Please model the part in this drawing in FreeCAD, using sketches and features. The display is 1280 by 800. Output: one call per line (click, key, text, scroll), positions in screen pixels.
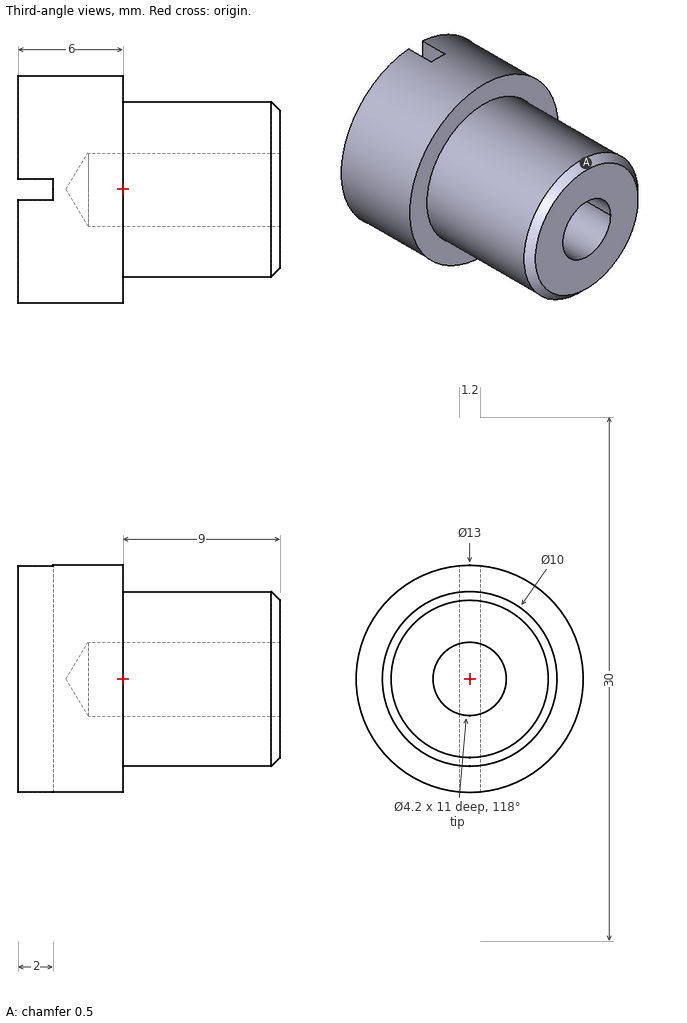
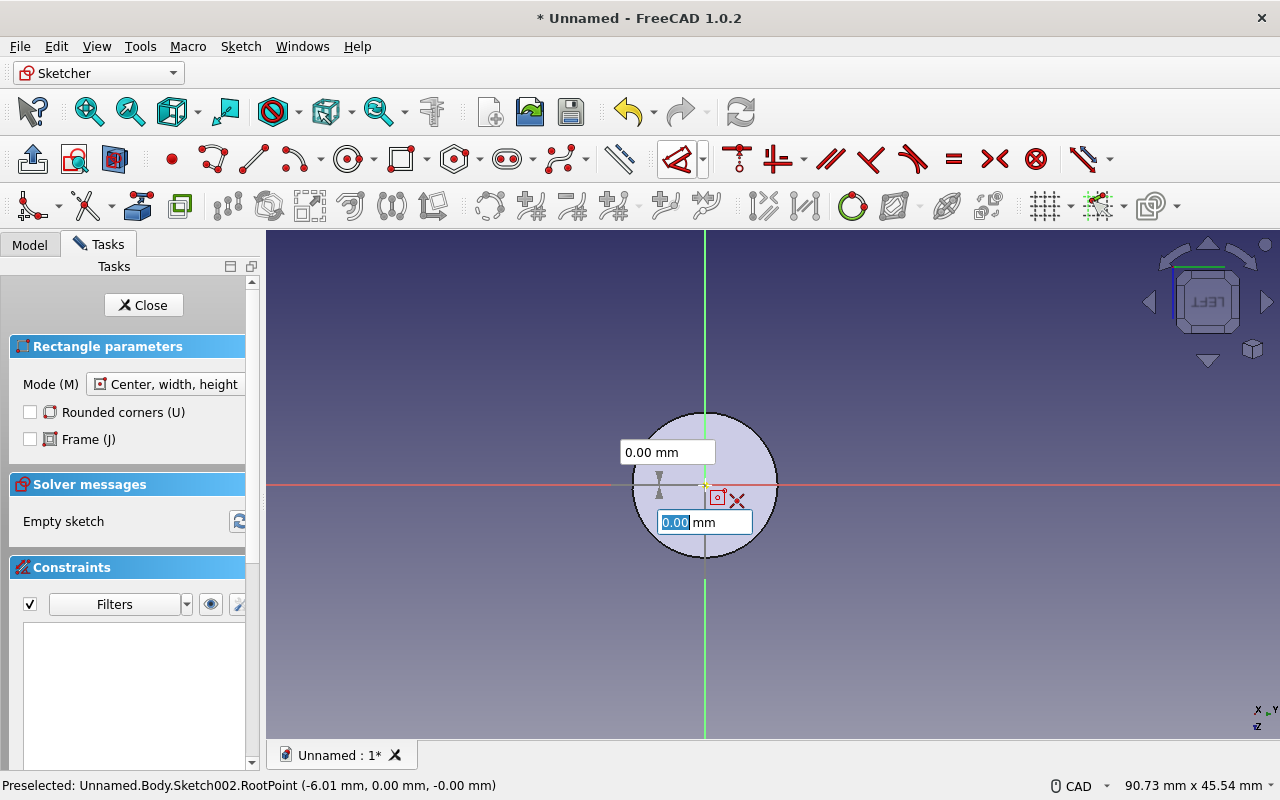
scroll(712, 317, up, 5)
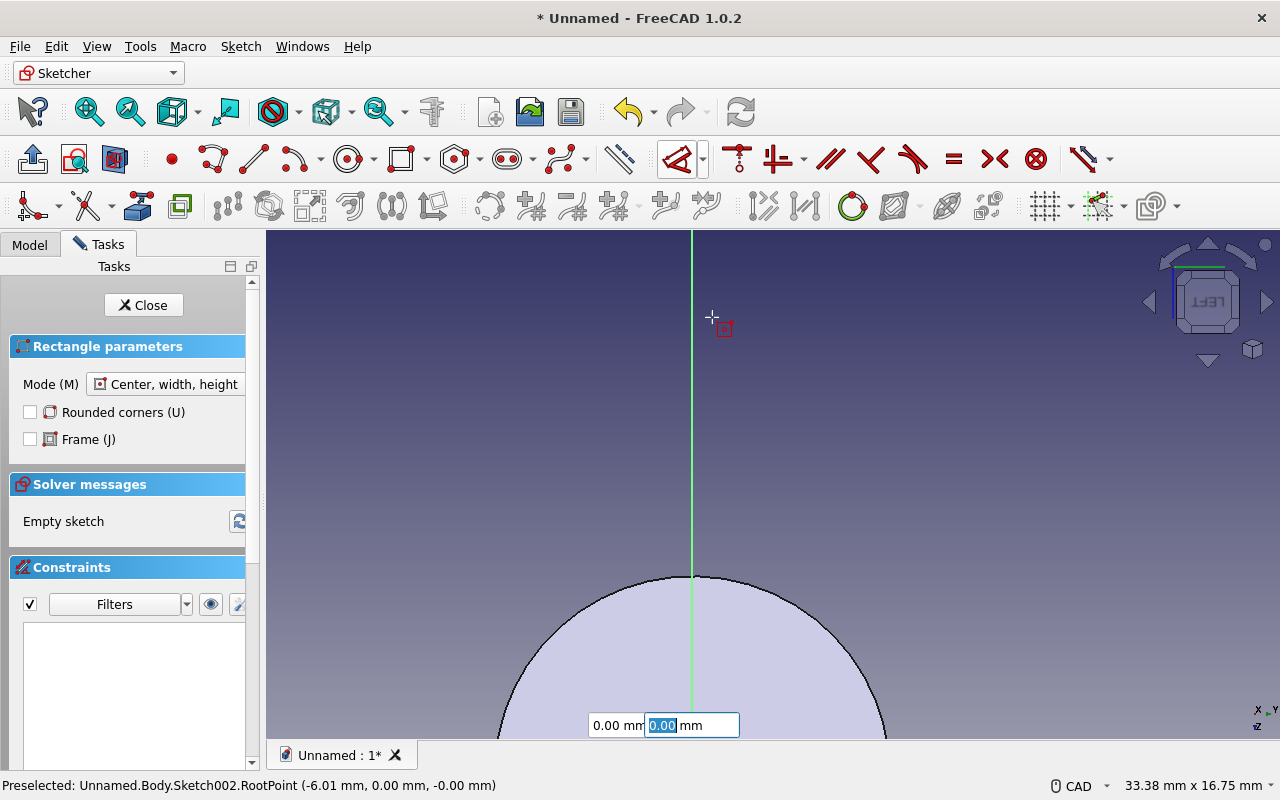
click(710, 318)
key(Escape)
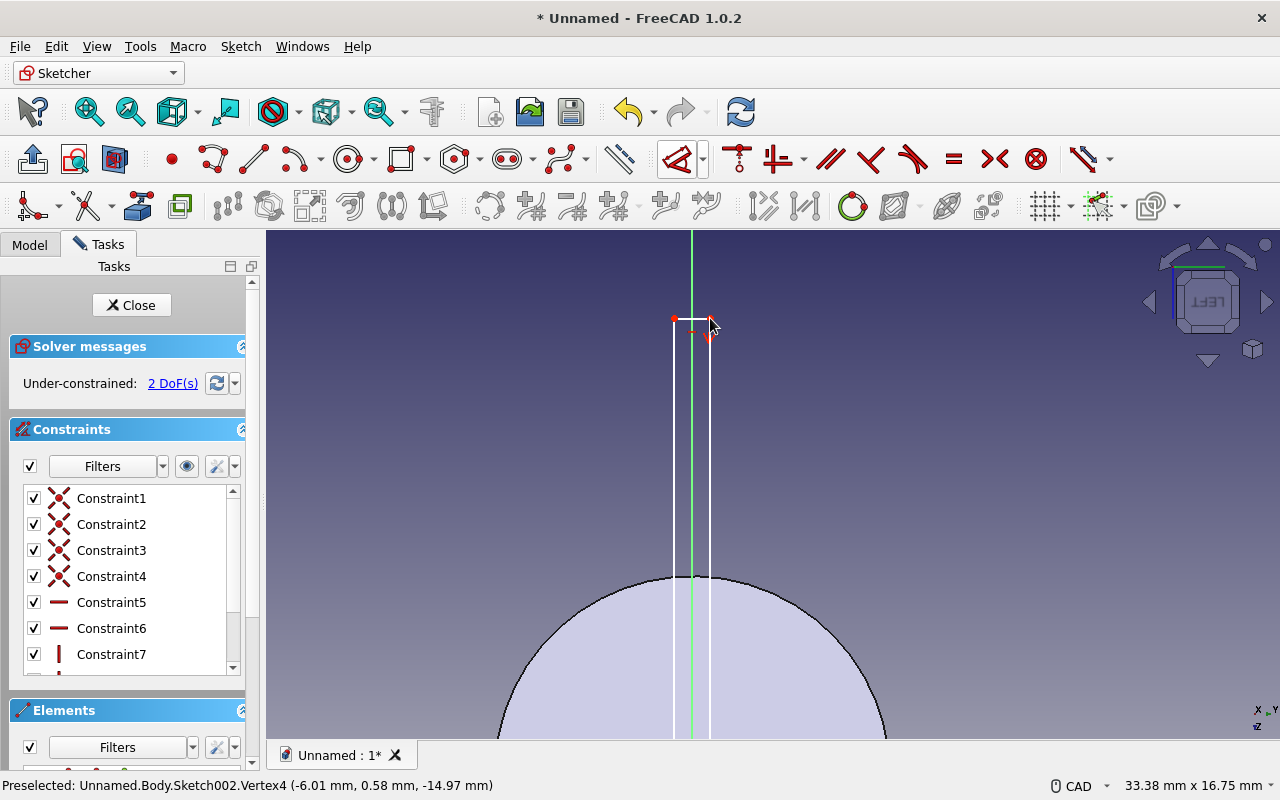
click(676, 160)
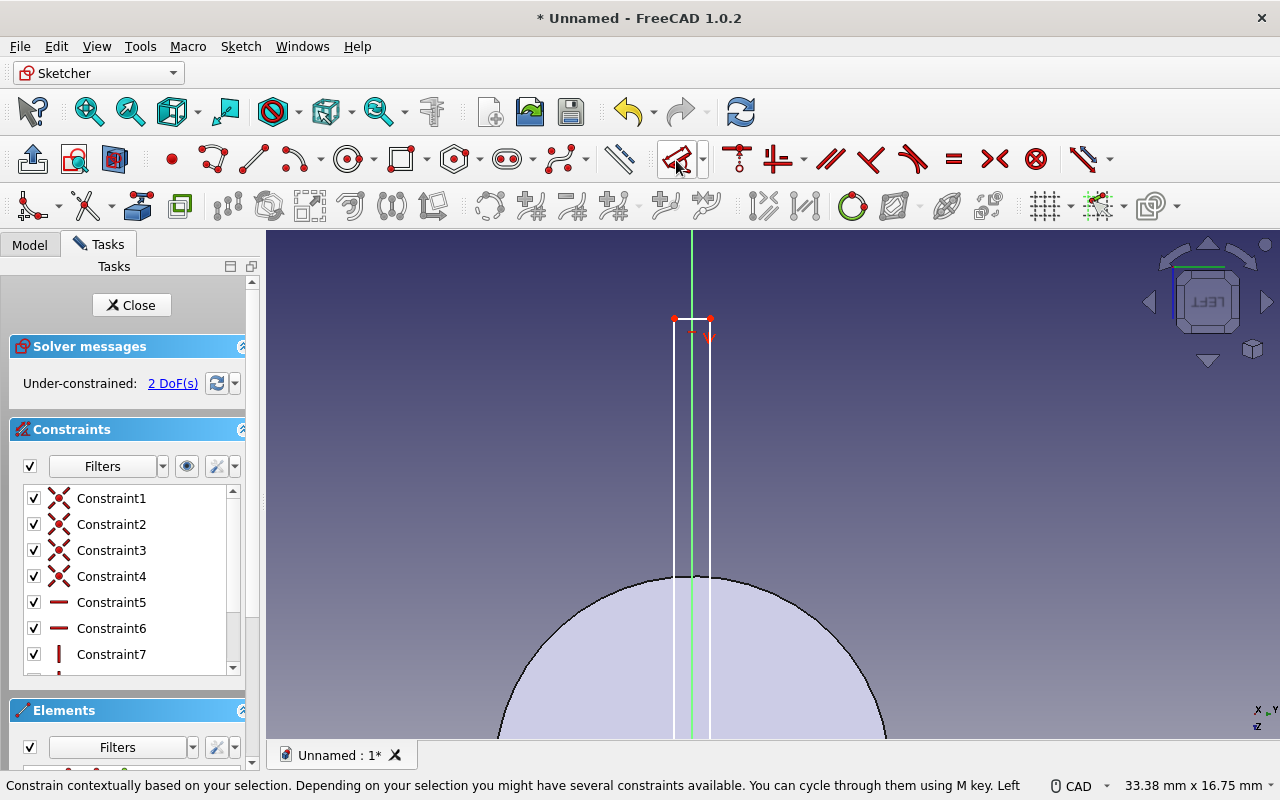
click(710, 592)
click(744, 515)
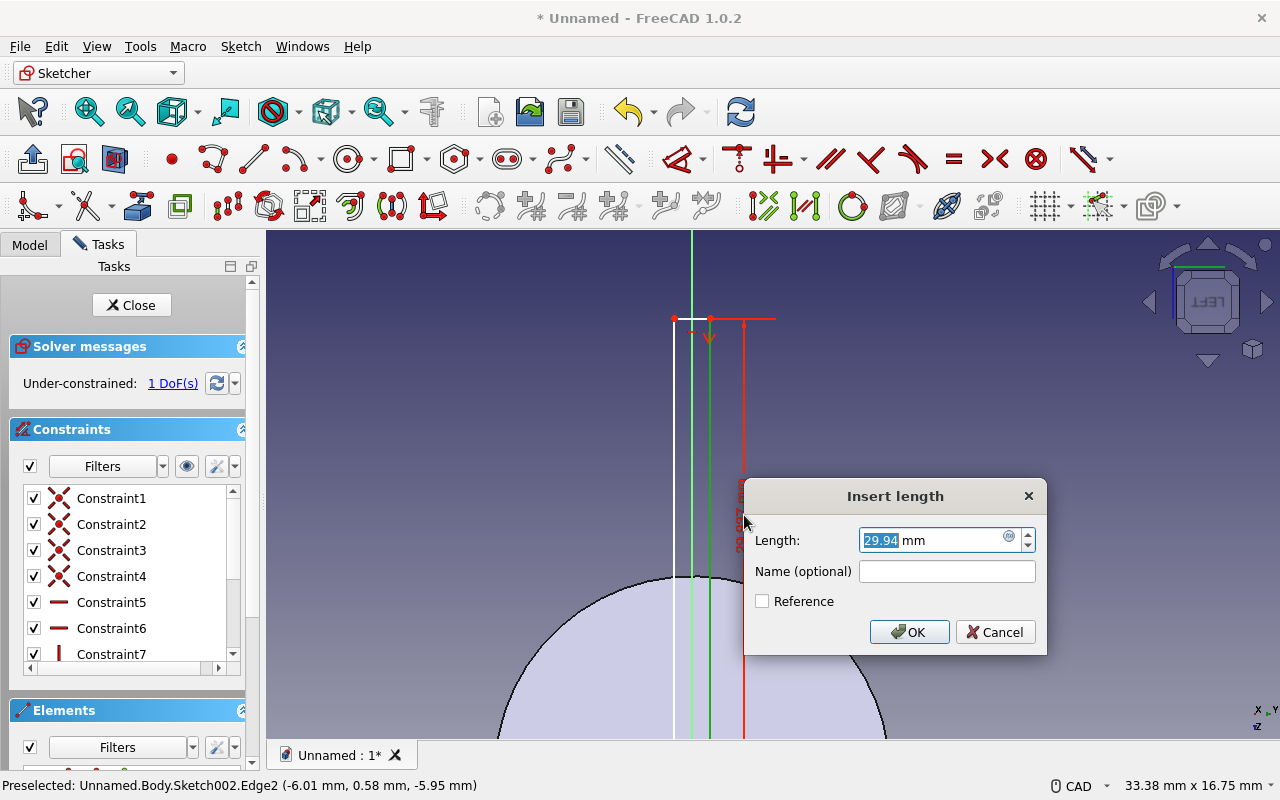
text(30)
key(Return)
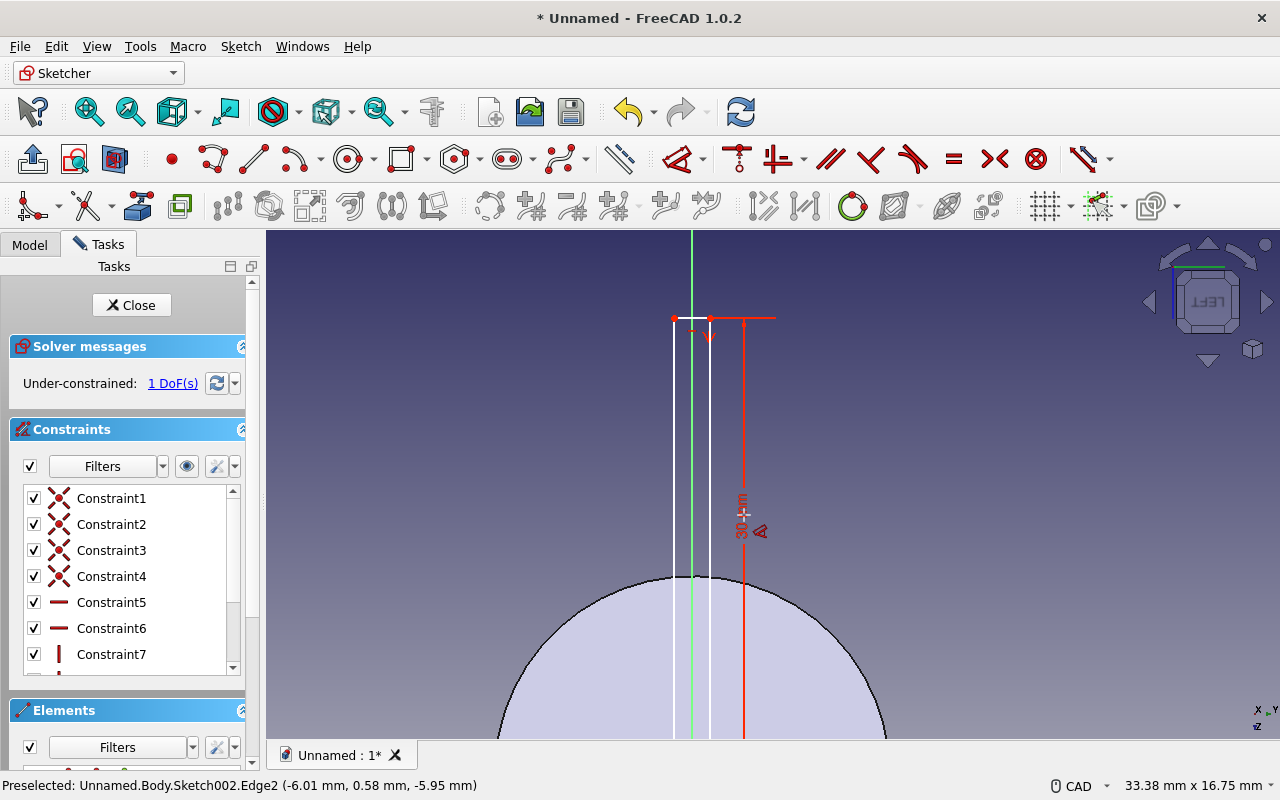
scroll(712, 316, down, 5)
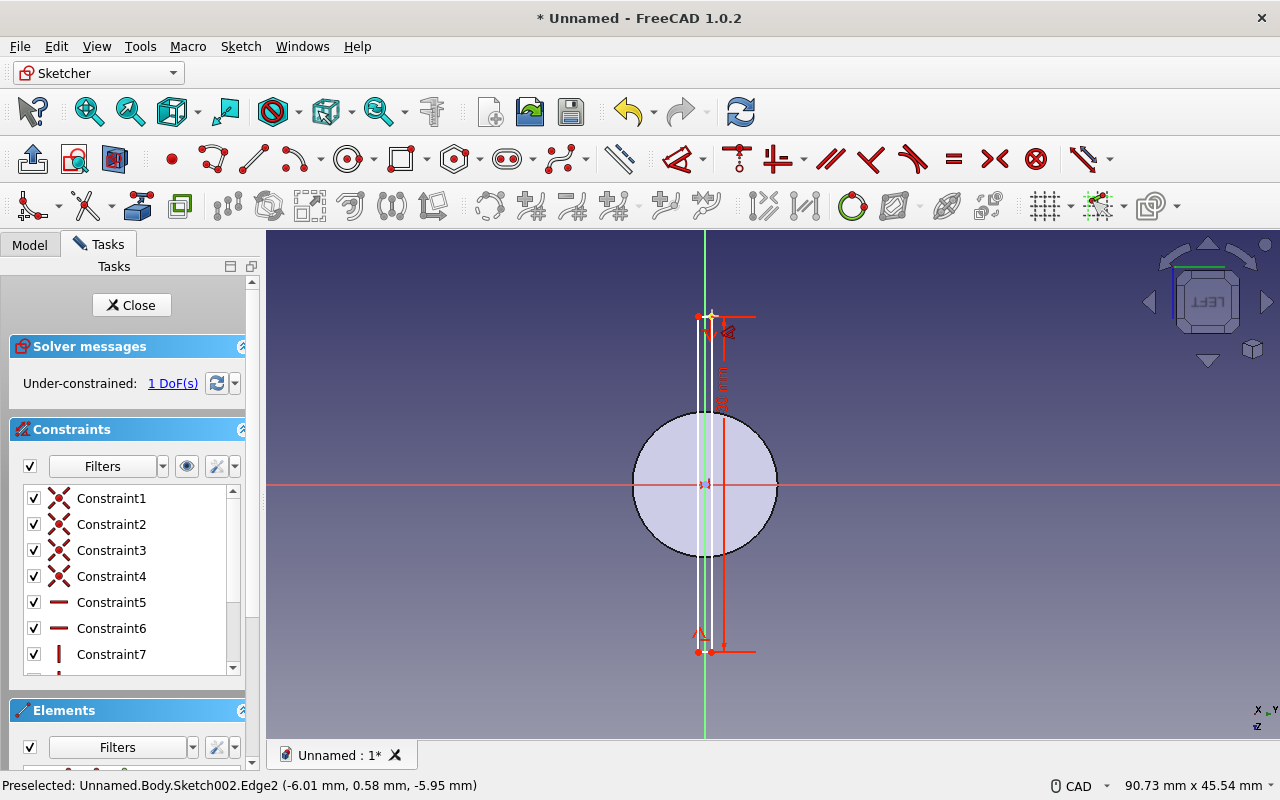
scroll(704, 652, up, 6)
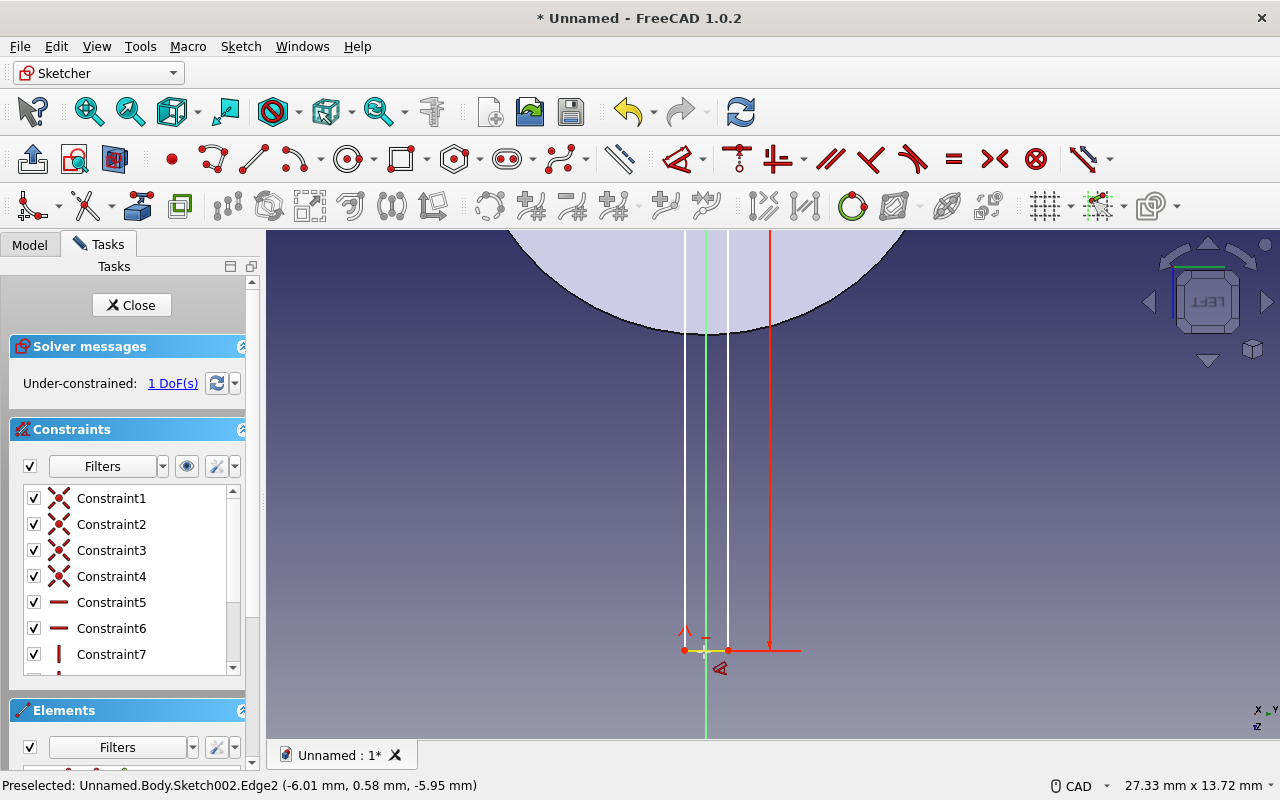
click(702, 651)
click(691, 685)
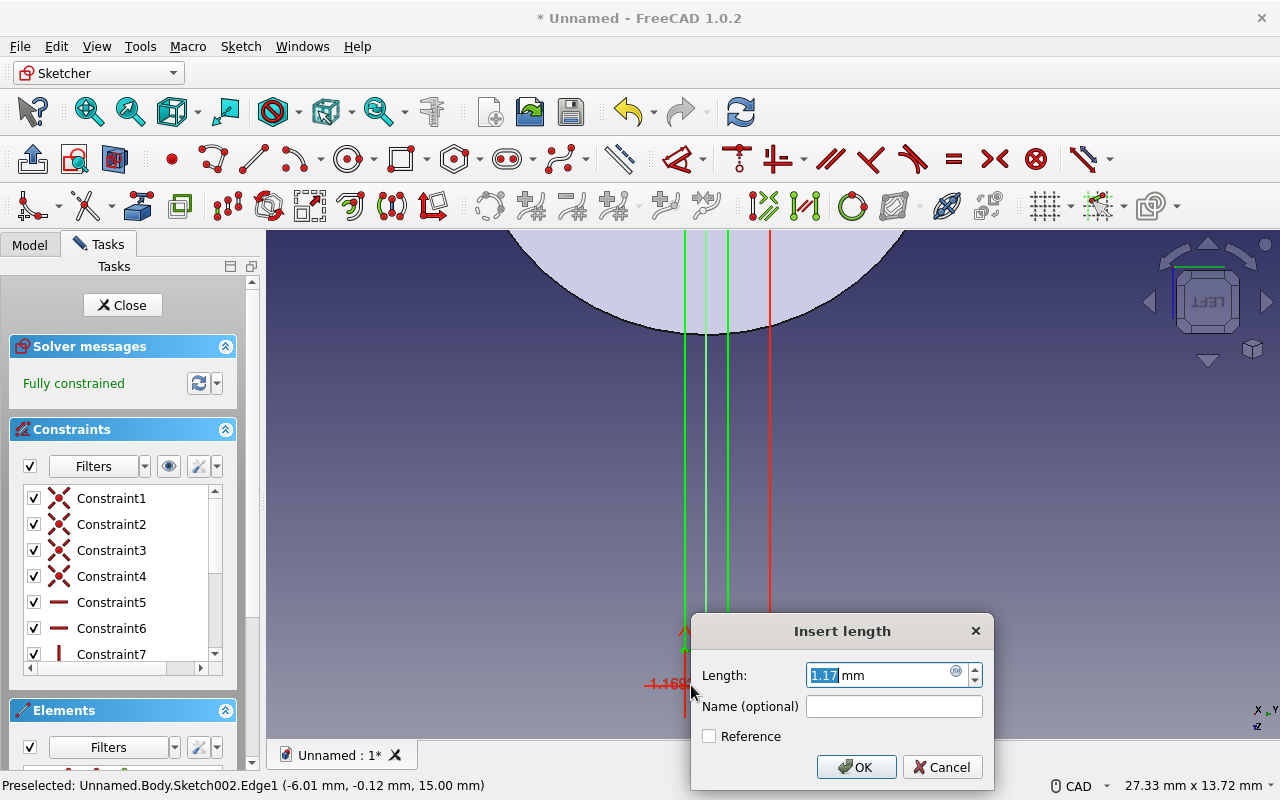
text(1.2)
key(Return)
key(Escape)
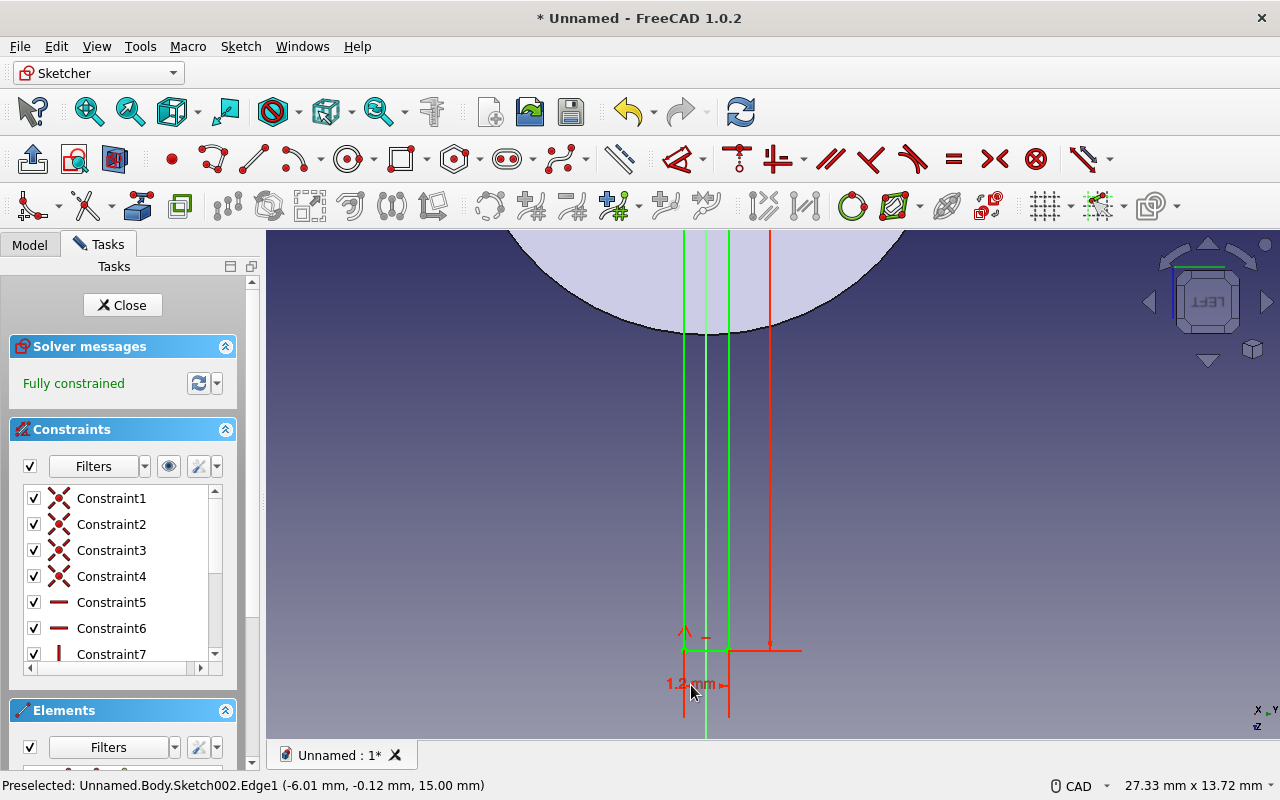
click(123, 305)